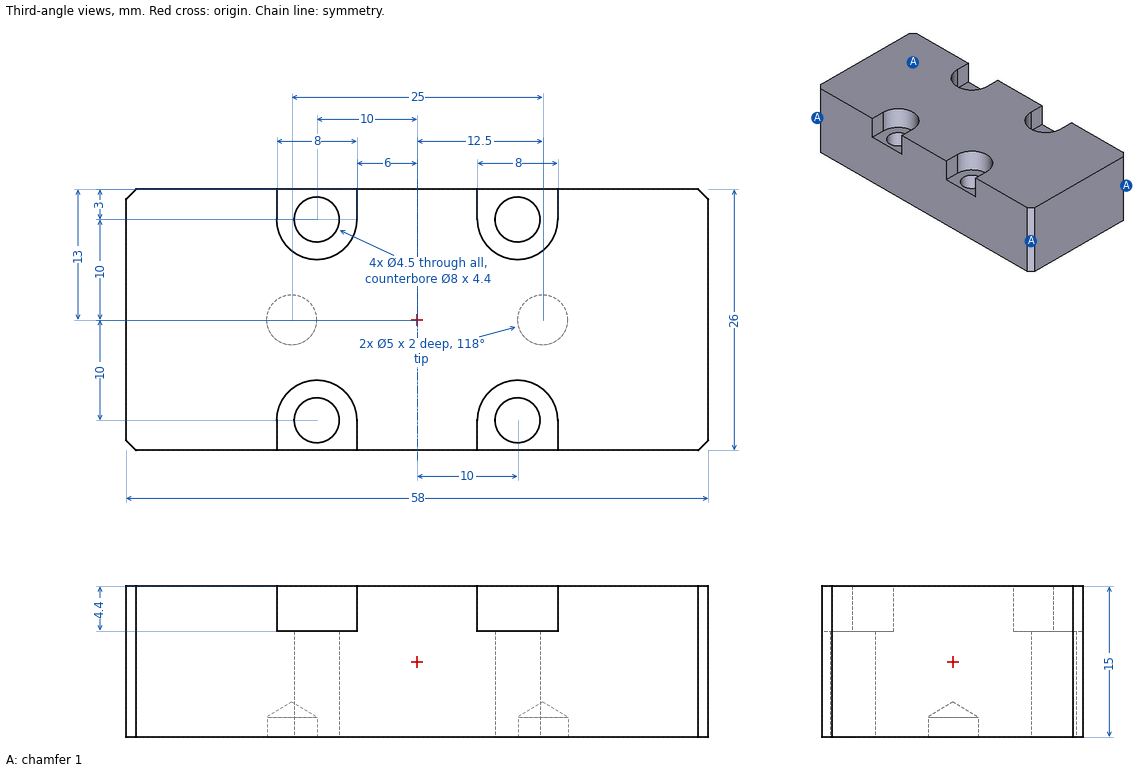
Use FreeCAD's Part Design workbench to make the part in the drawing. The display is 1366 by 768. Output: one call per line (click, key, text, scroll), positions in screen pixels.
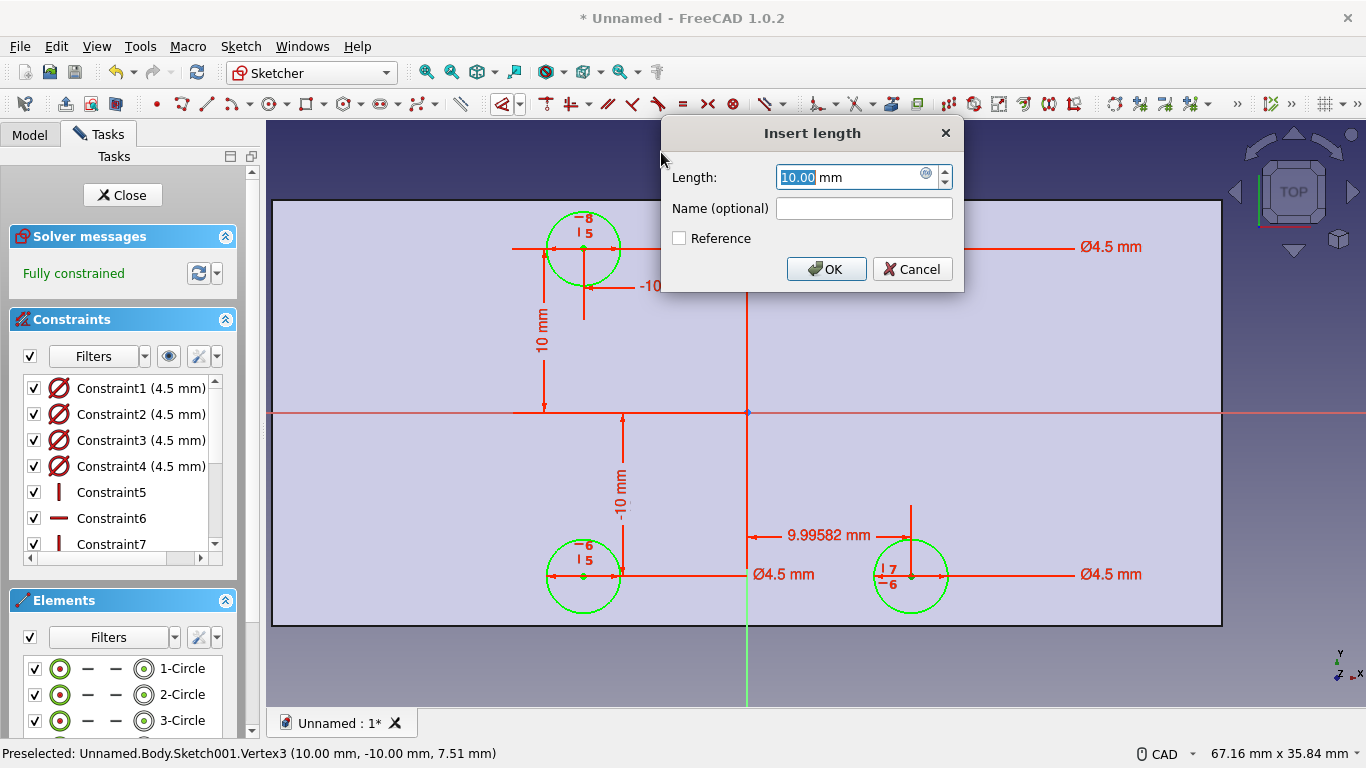
text(10)
key(Return)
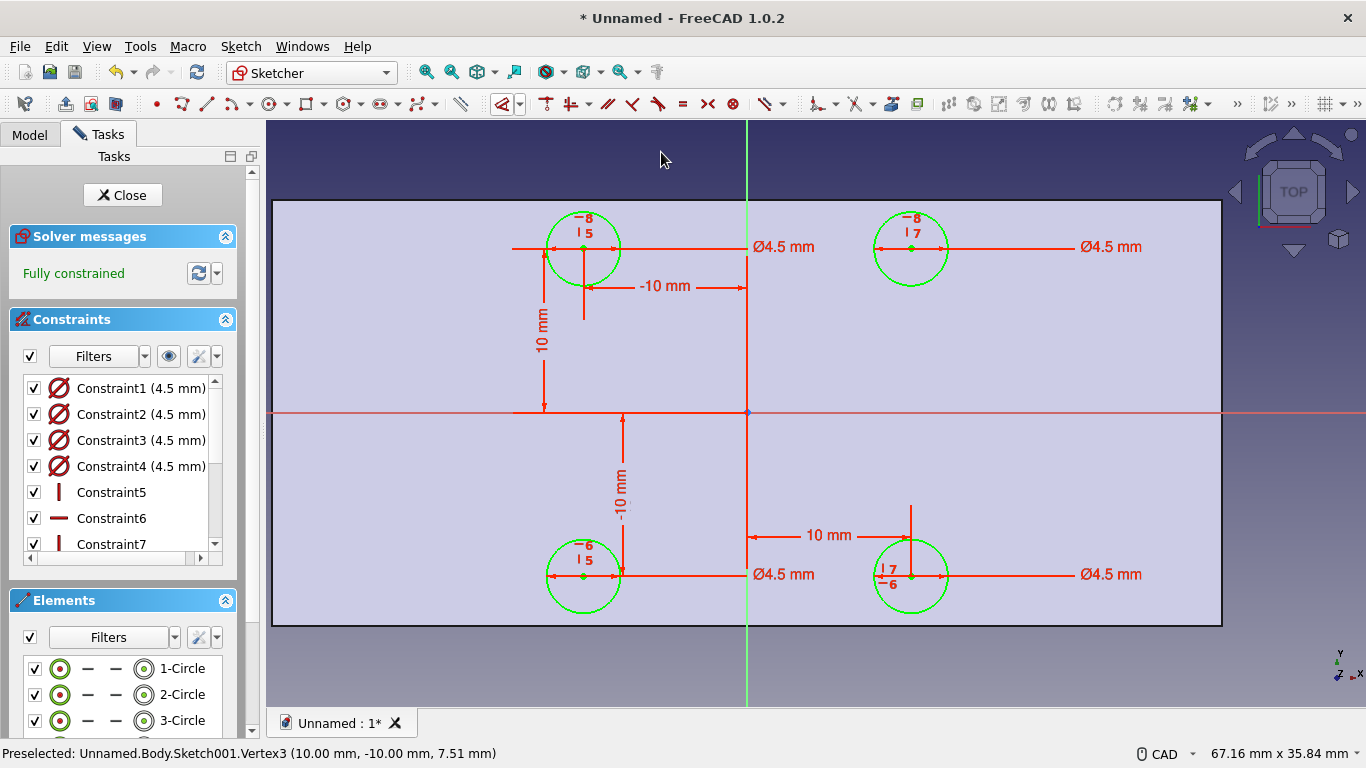
click(123, 195)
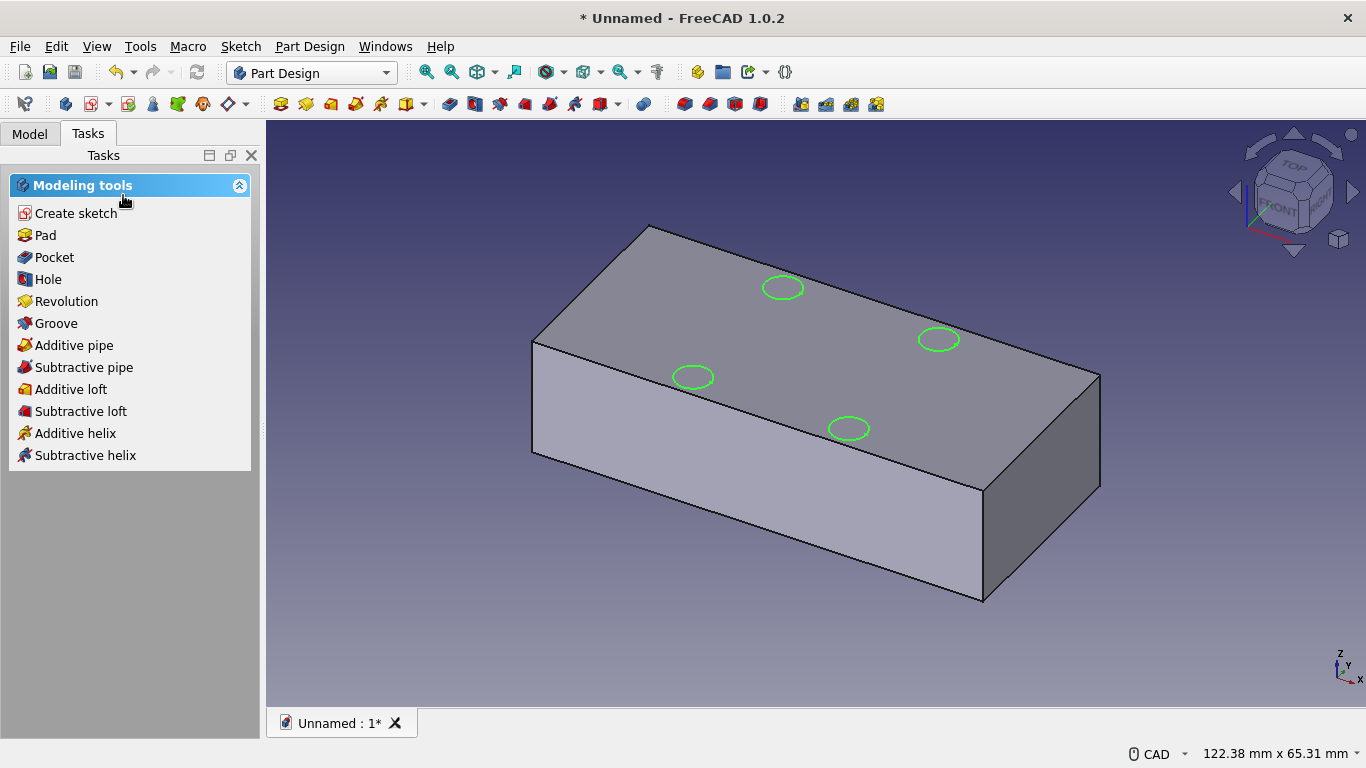
click(475, 104)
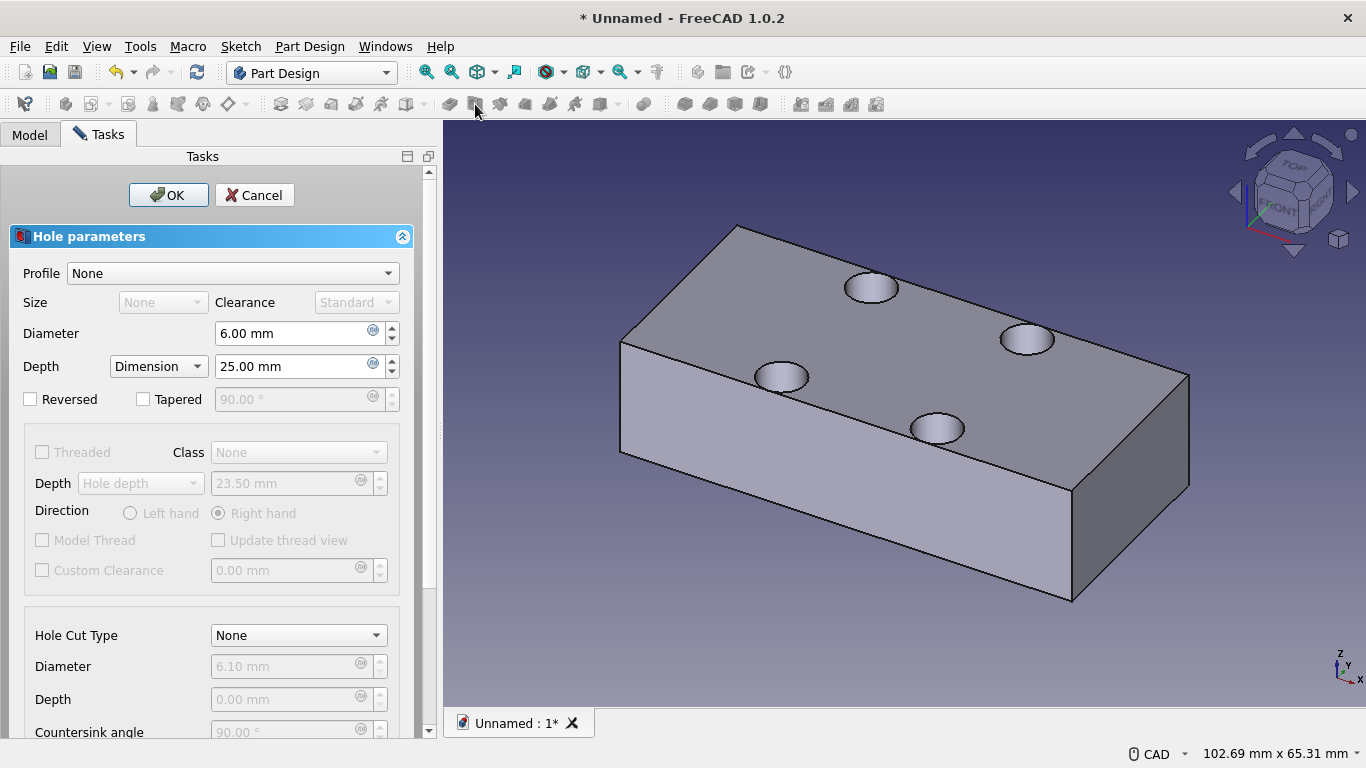
triple_click(300, 334)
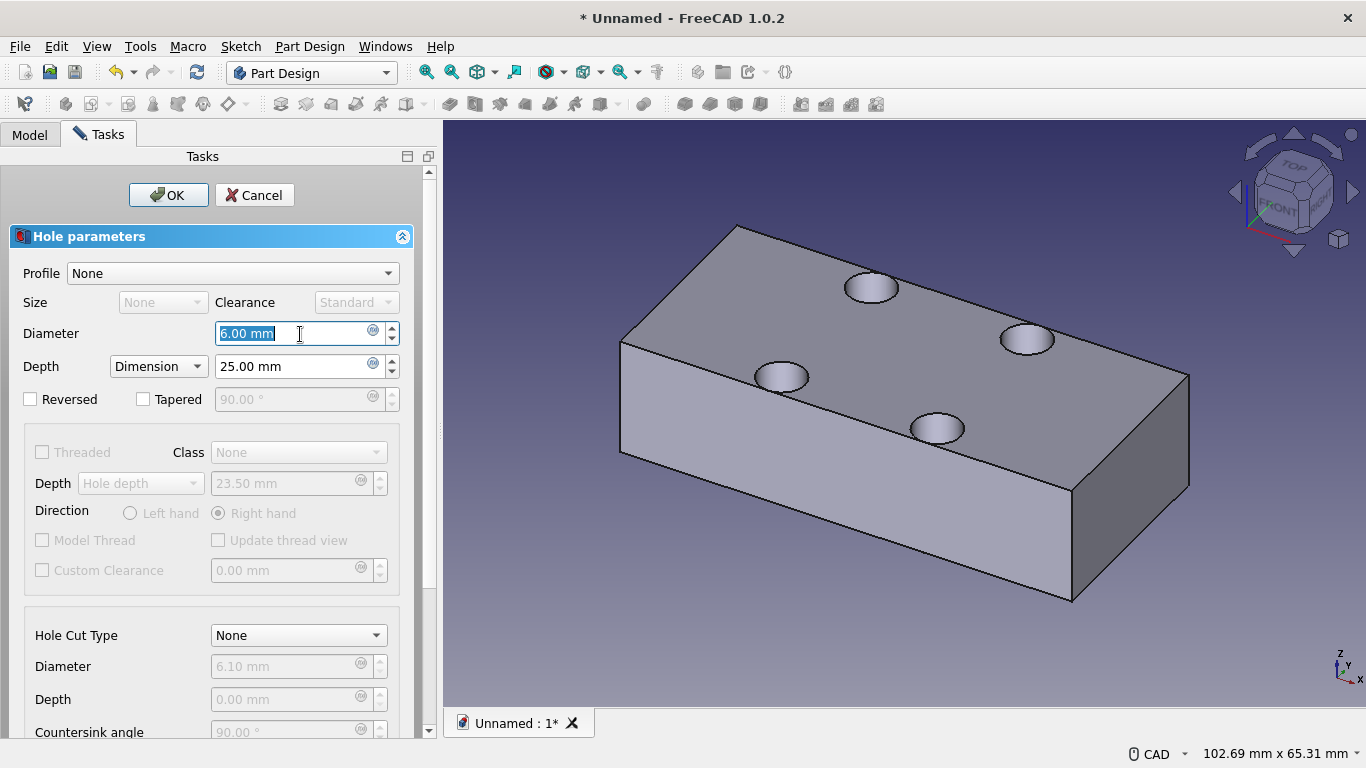
text(4.5)
key(Tab)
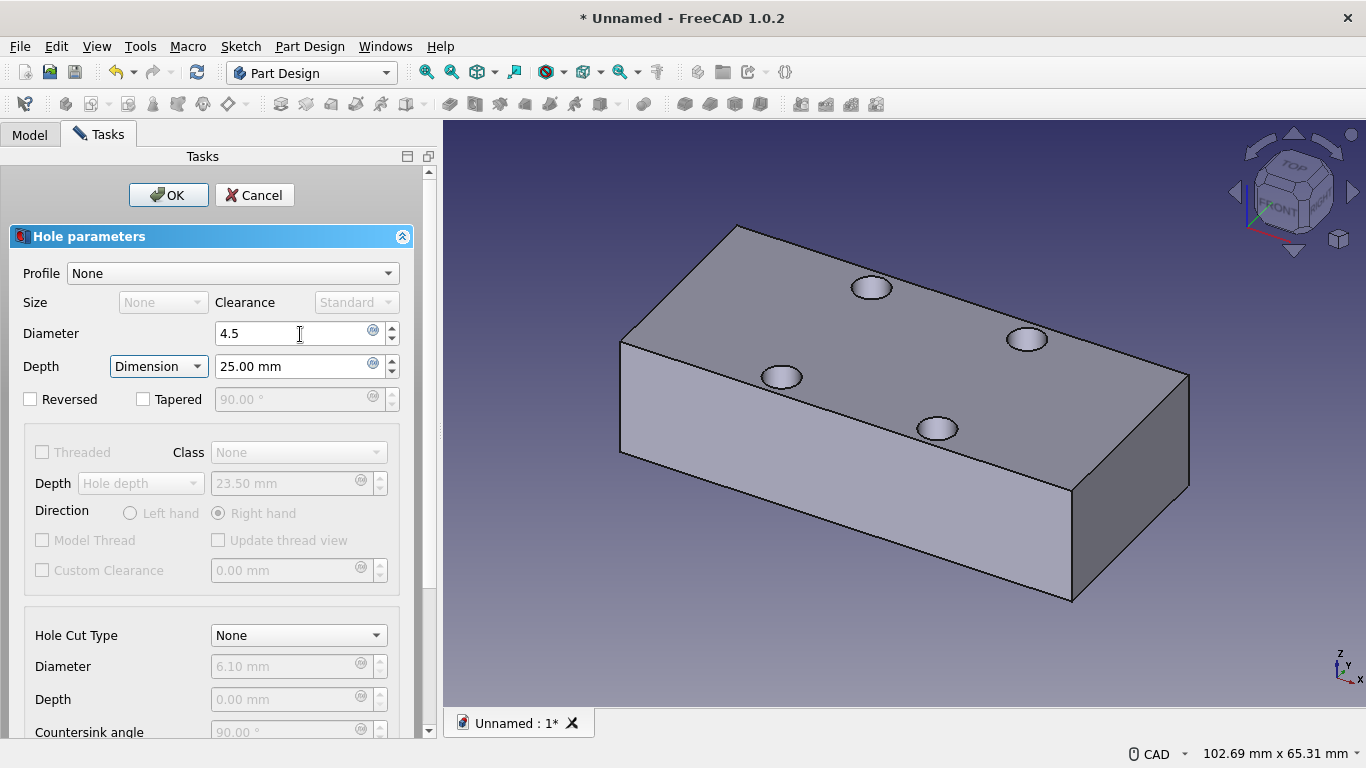
click(160, 366)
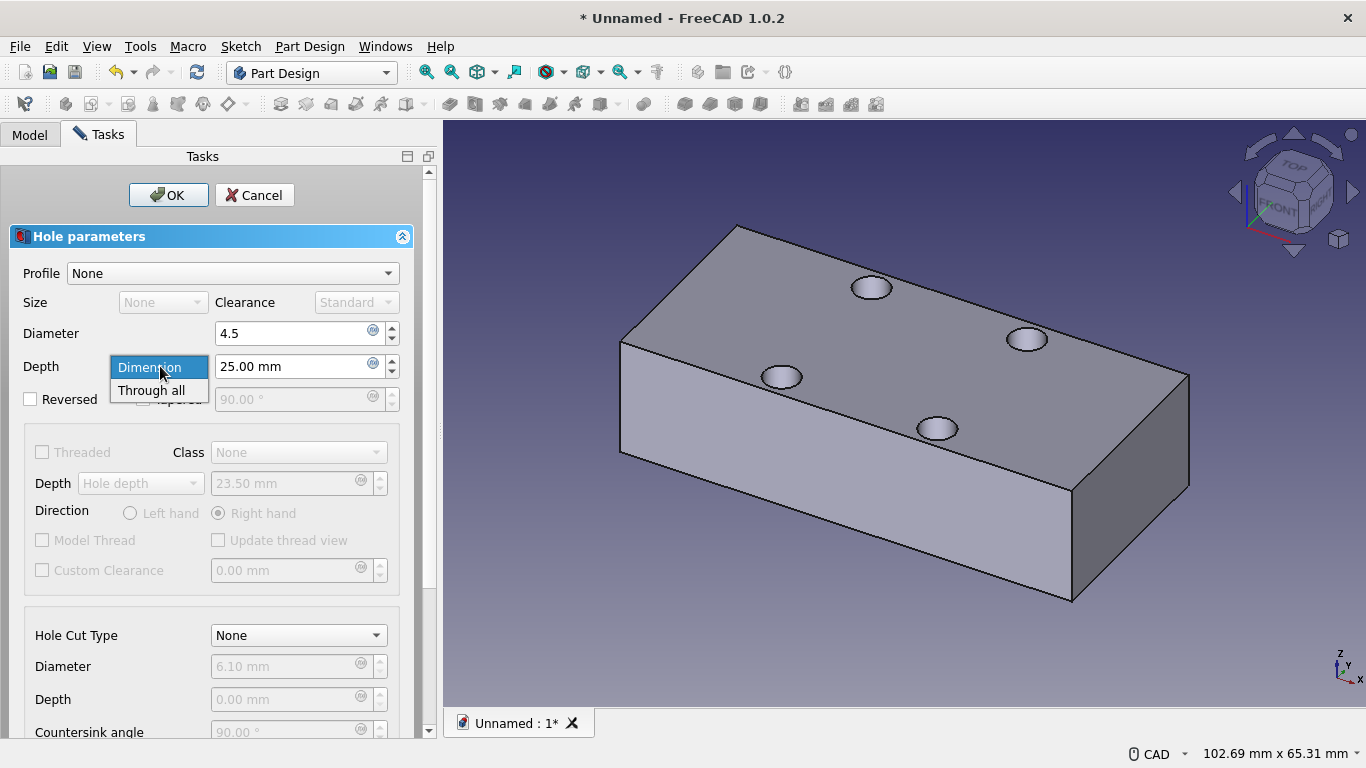
click(158, 390)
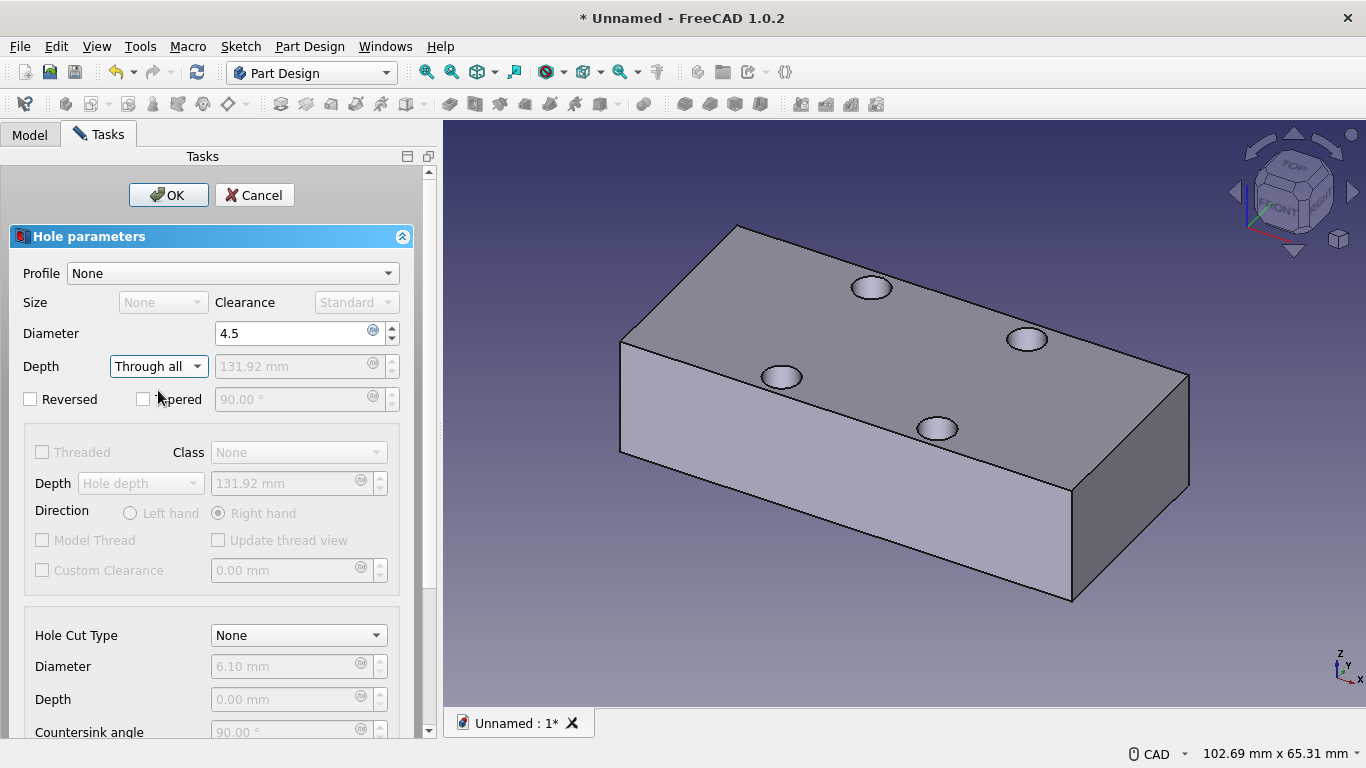
click(300, 636)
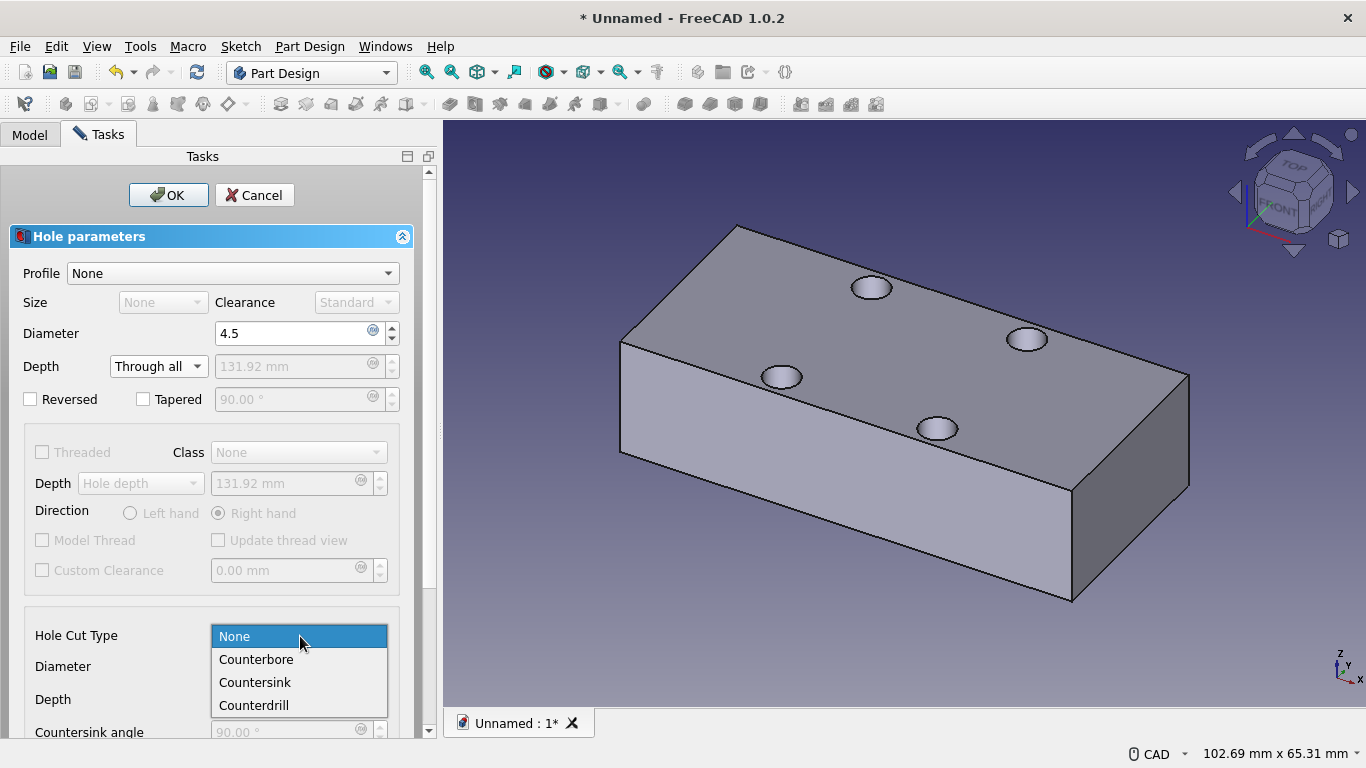
click(298, 660)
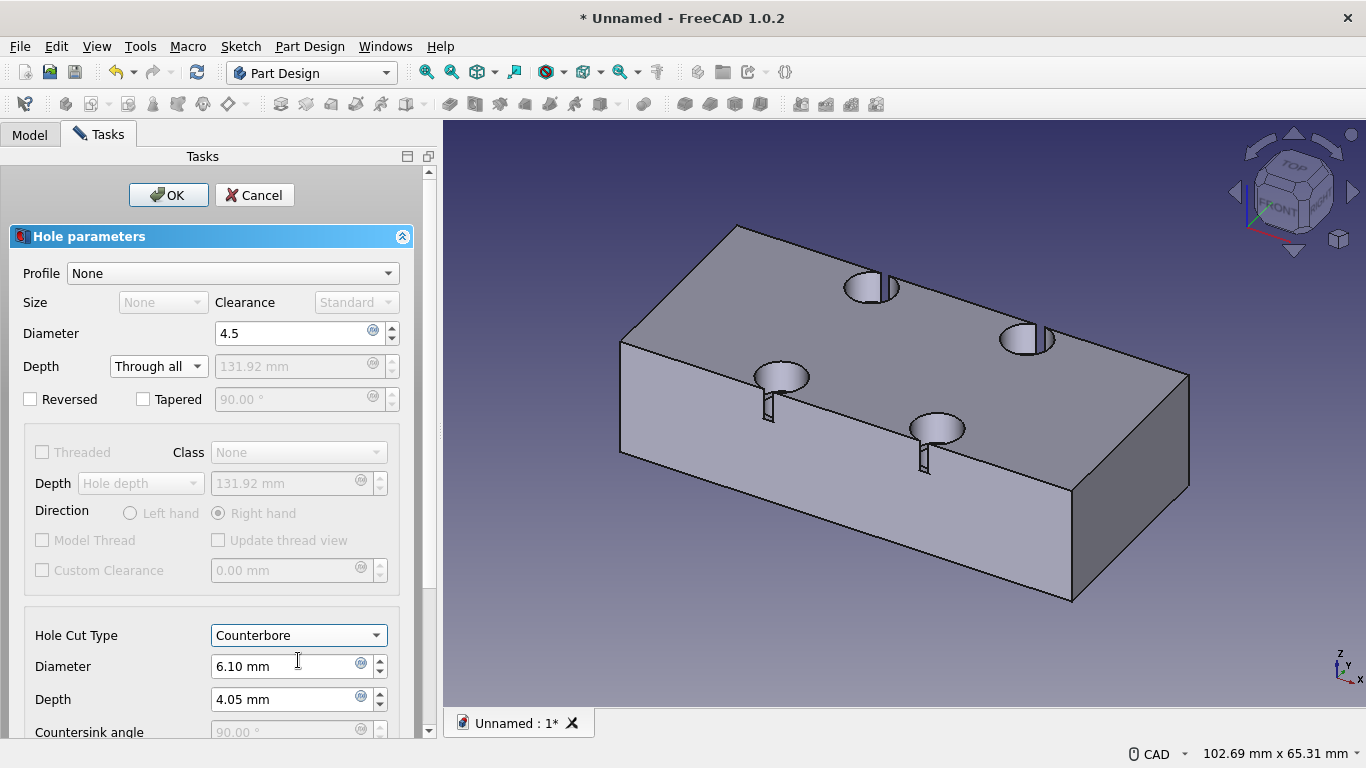
triple_click(292, 666)